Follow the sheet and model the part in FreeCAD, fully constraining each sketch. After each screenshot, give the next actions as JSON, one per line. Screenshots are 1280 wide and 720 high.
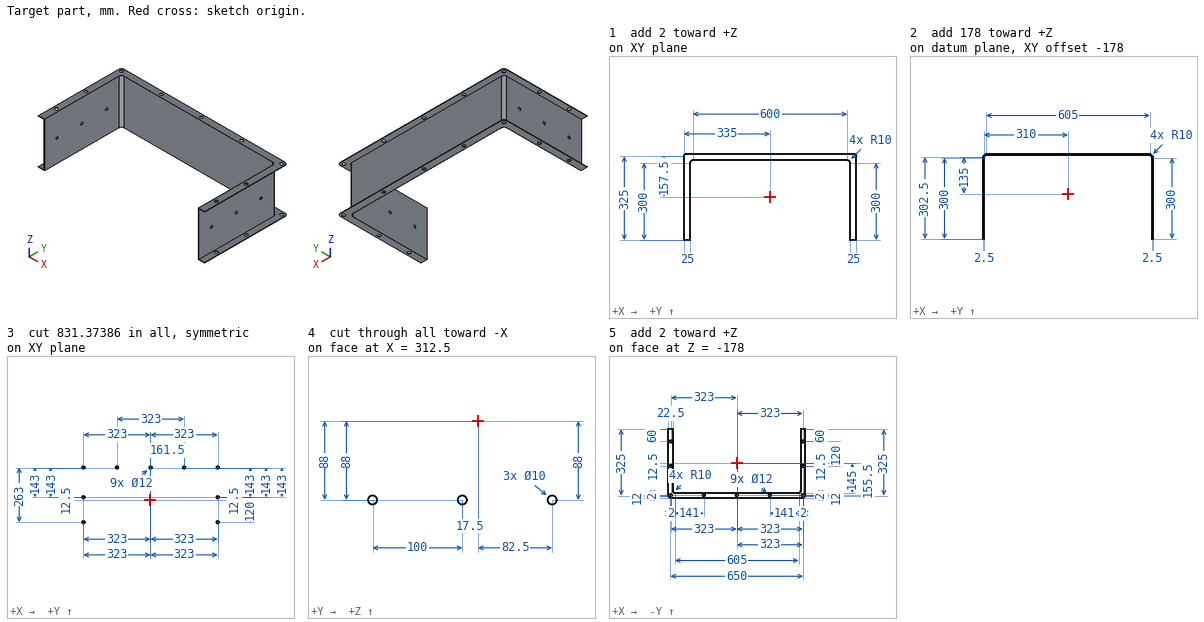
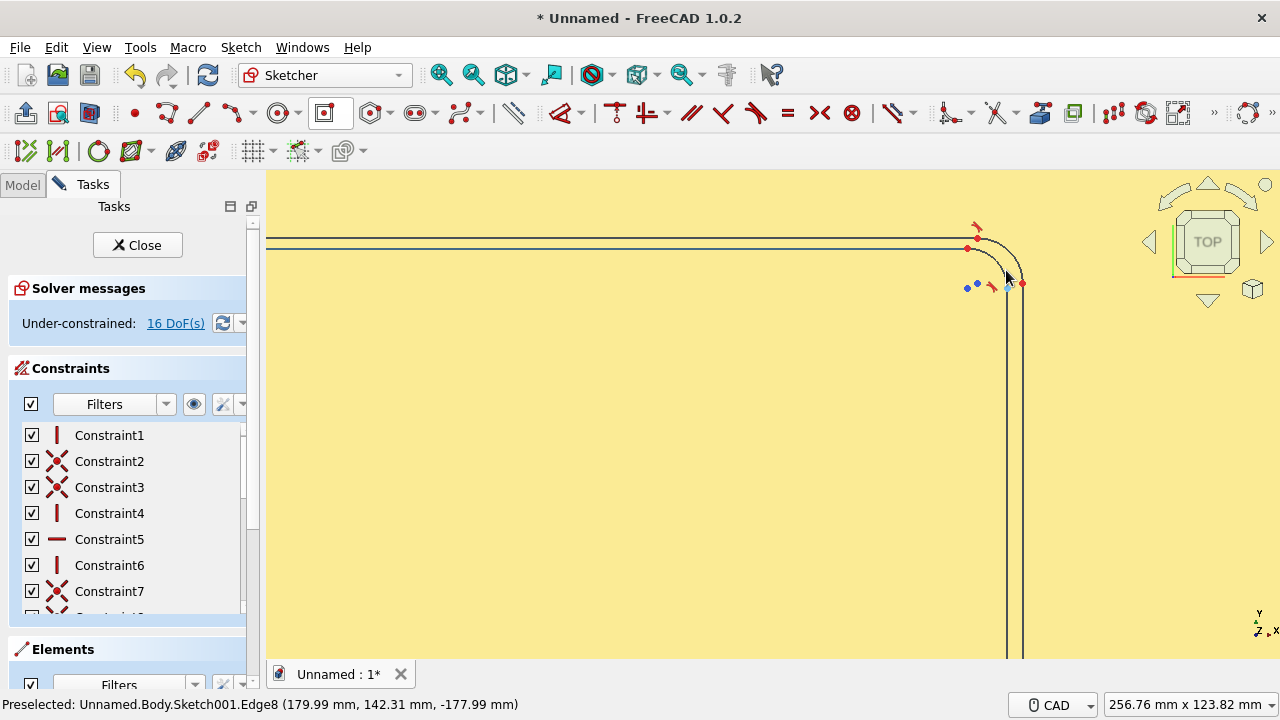
{"action": "left_click", "coordinate": [1003, 270]}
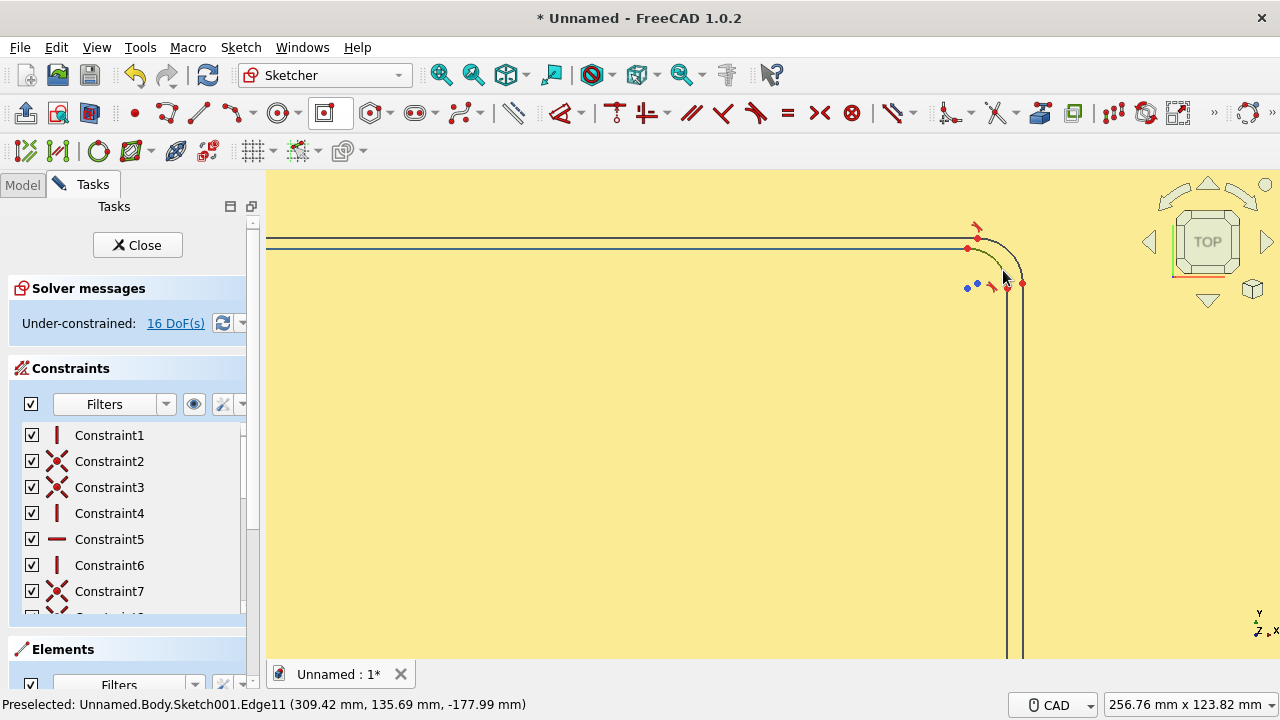
{"action": "left_click", "coordinate": [756, 114]}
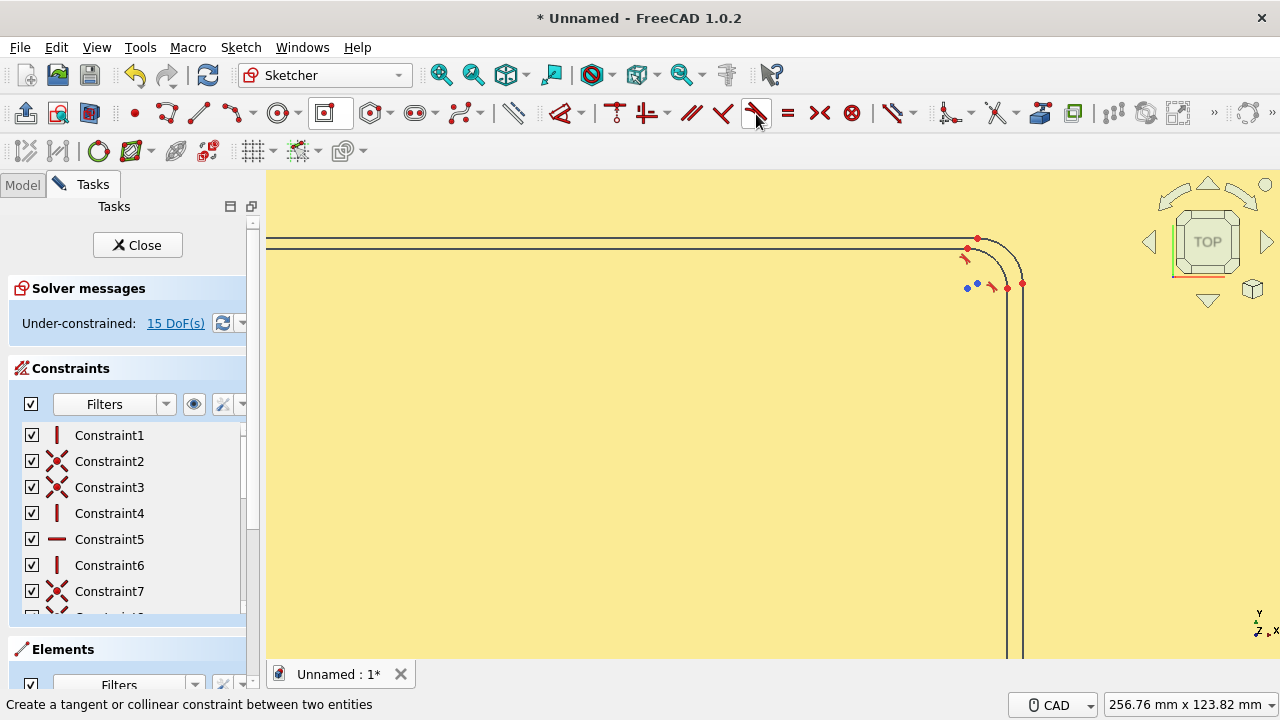
{"action": "scroll", "coordinate": [494, 249], "scroll_direction": "up", "scroll_amount": 2}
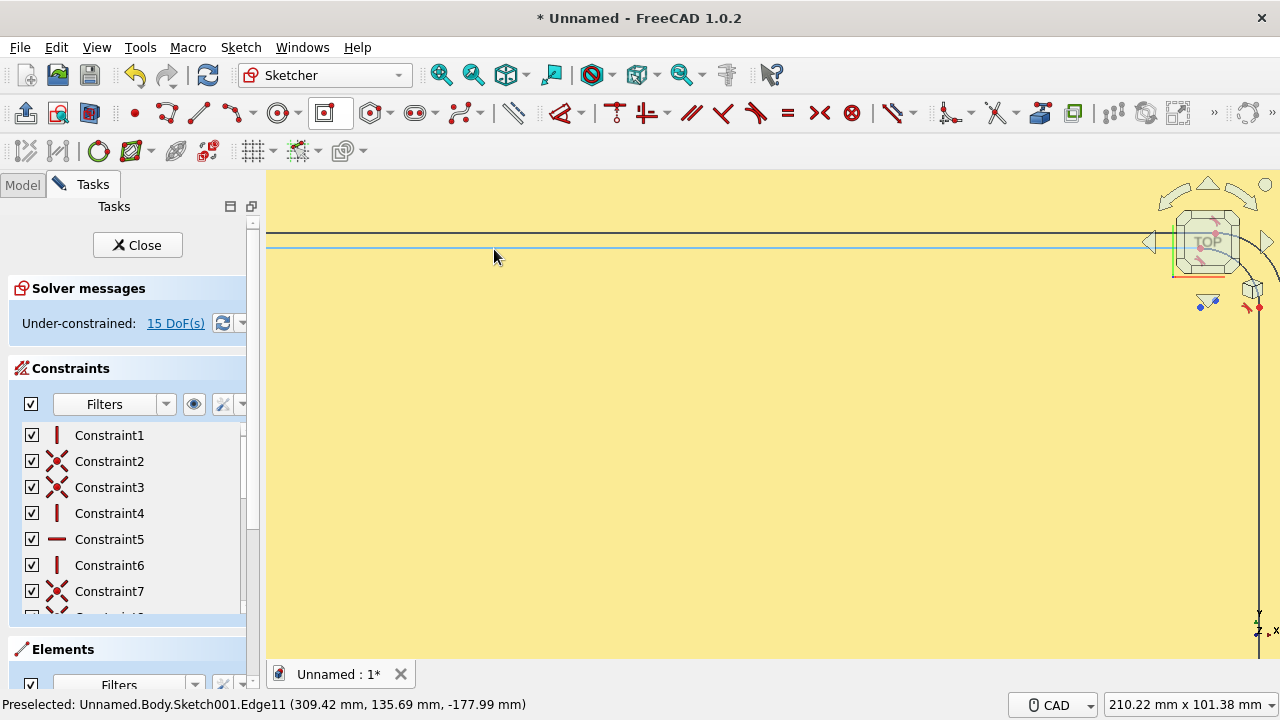
{"action": "left_click", "coordinate": [493, 248]}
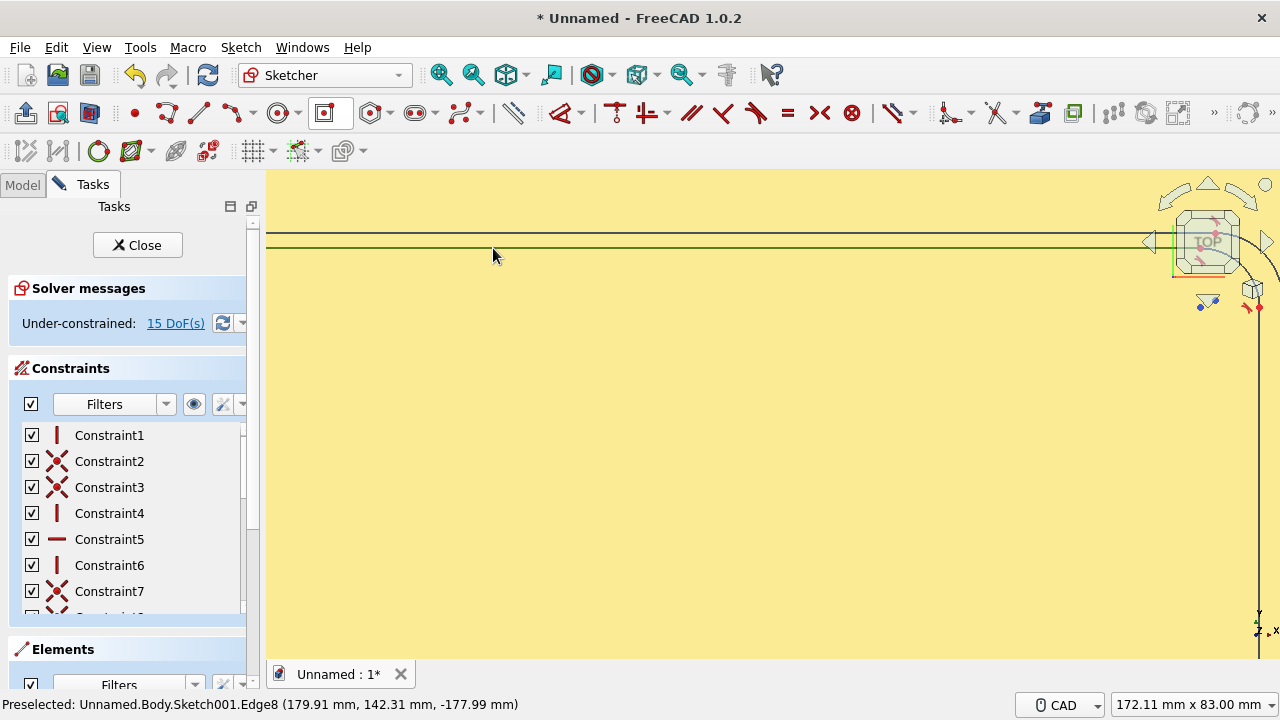
{"action": "scroll", "coordinate": [956, 268], "scroll_direction": "down", "scroll_amount": 9}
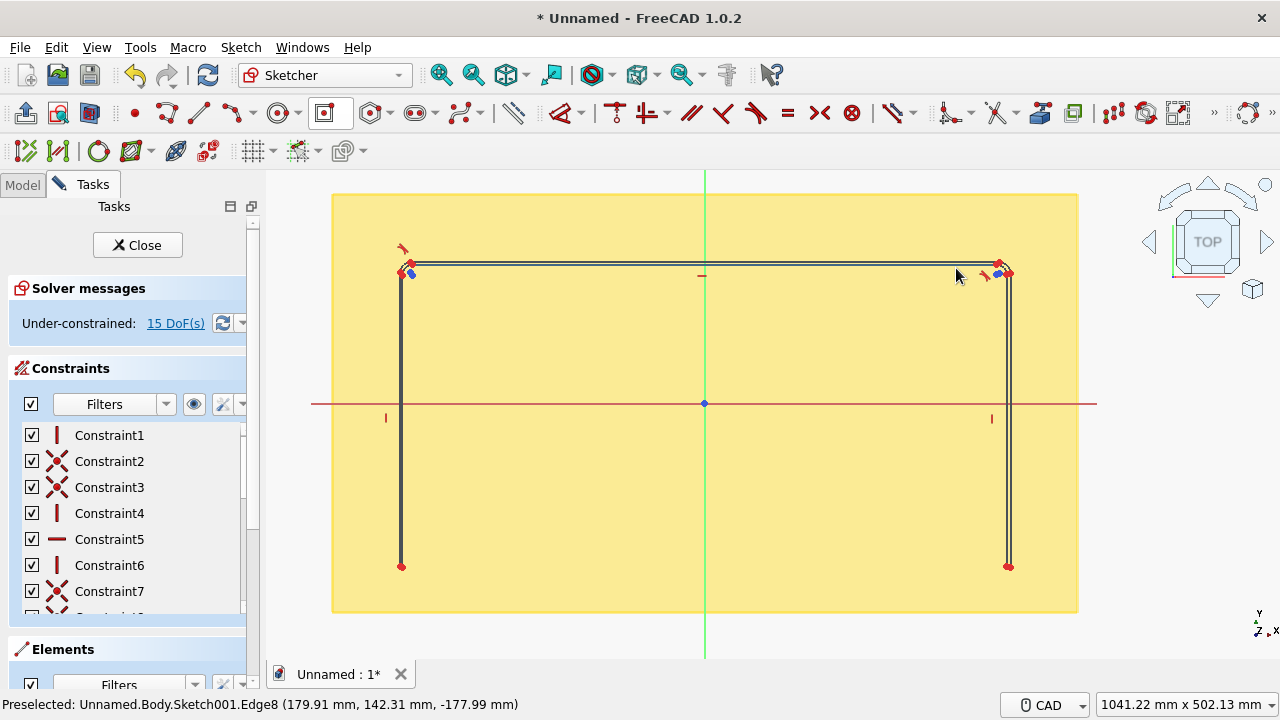
{"action": "scroll", "coordinate": [408, 266], "scroll_direction": "up", "scroll_amount": 8}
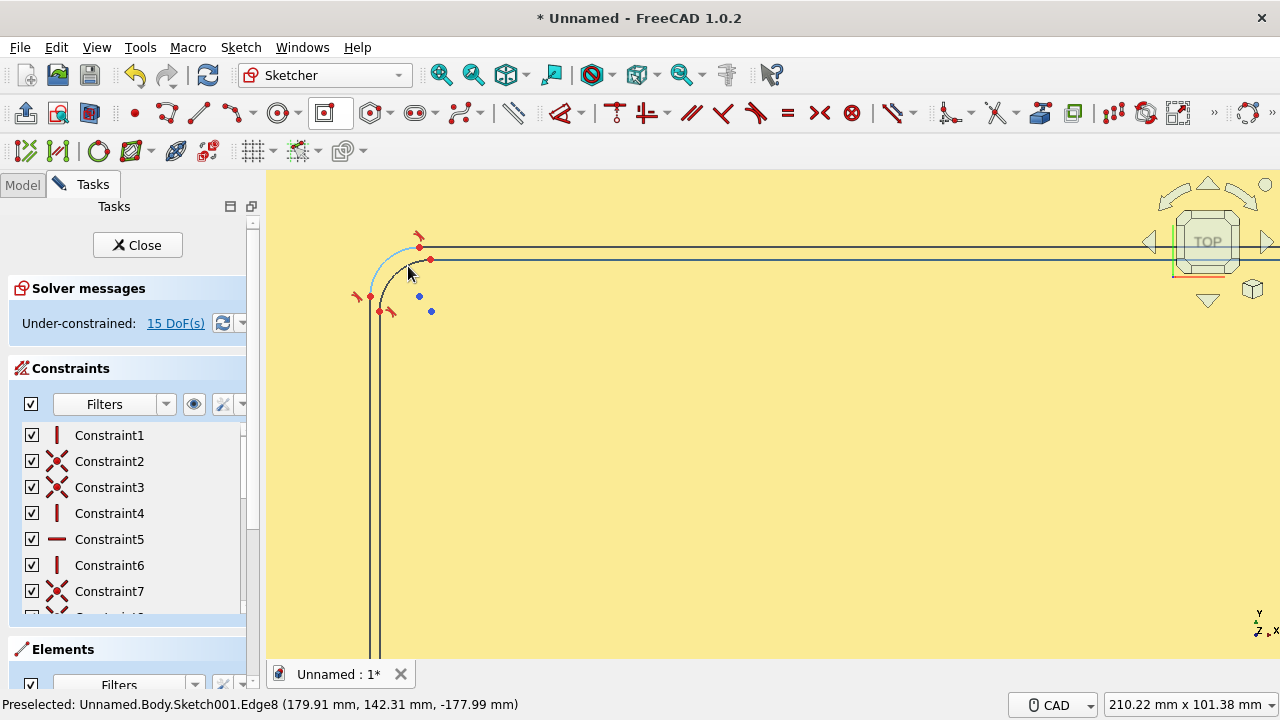
{"action": "left_click", "coordinate": [407, 266]}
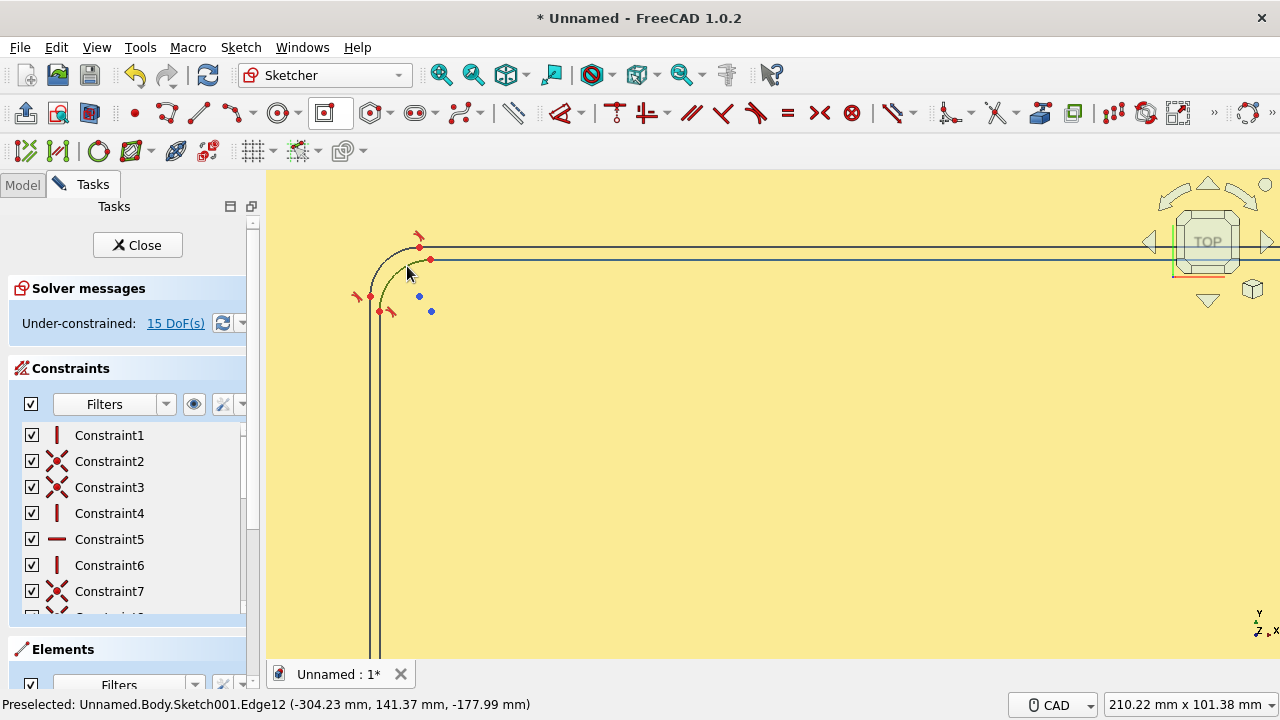
{"action": "left_click", "coordinate": [756, 114]}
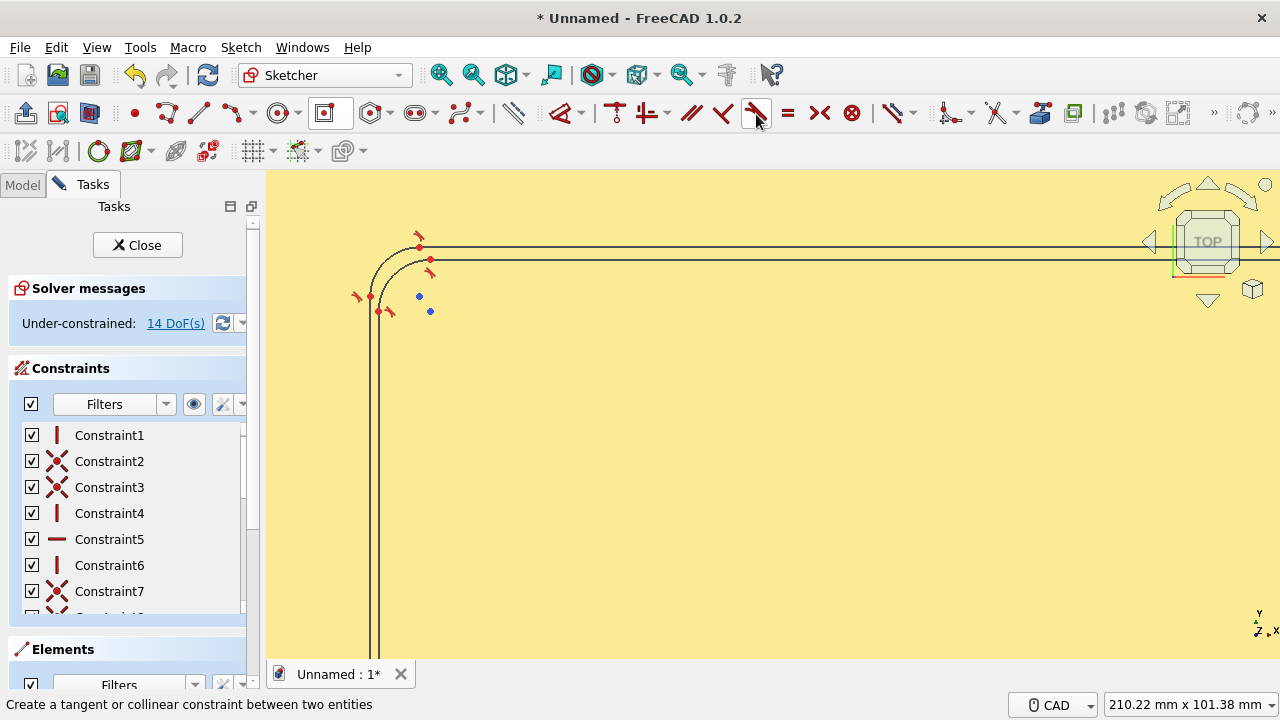
{"action": "scroll", "coordinate": [408, 266], "scroll_direction": "down", "scroll_amount": 8}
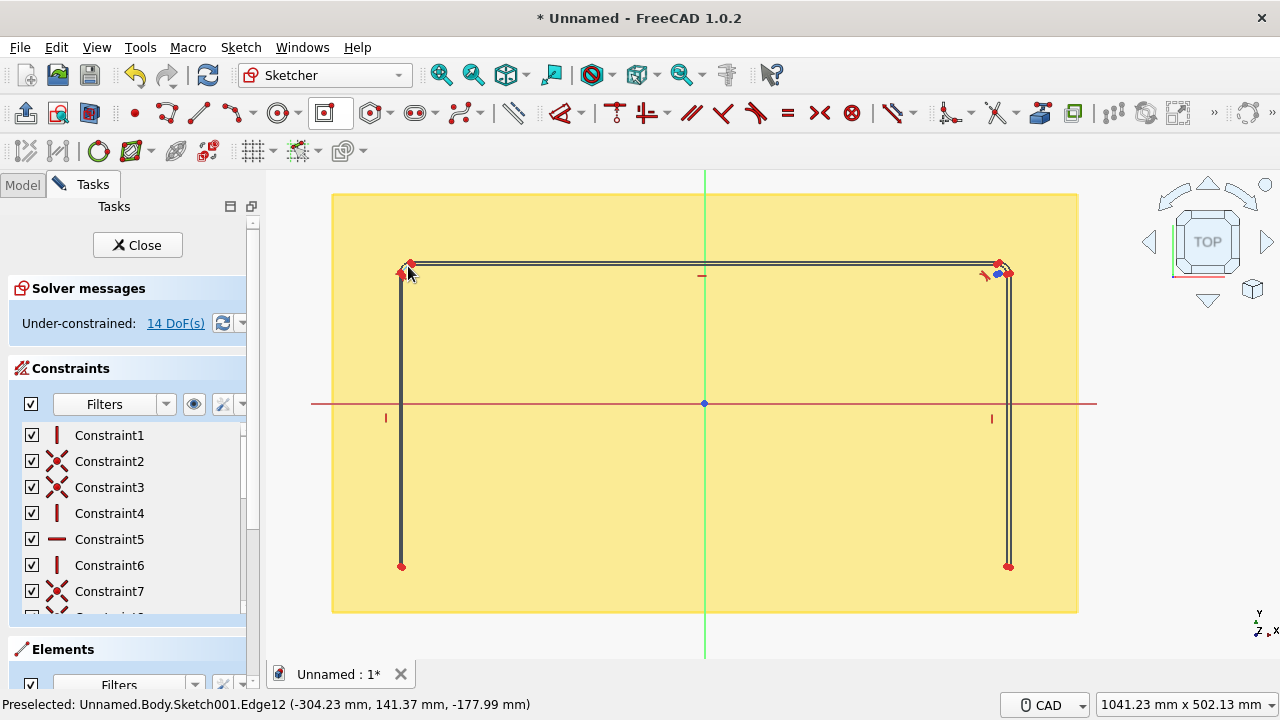
{"action": "scroll", "coordinate": [401, 567], "scroll_direction": "up", "scroll_amount": 14}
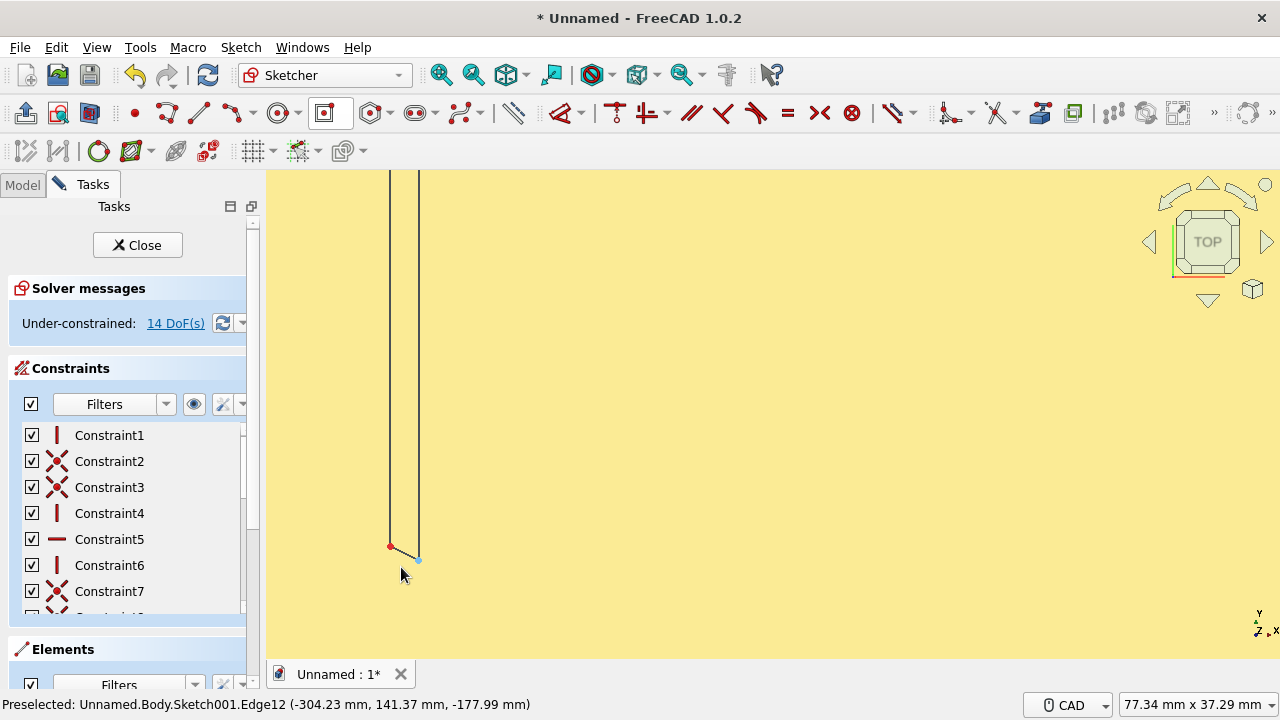
{"action": "left_click", "coordinate": [405, 553]}